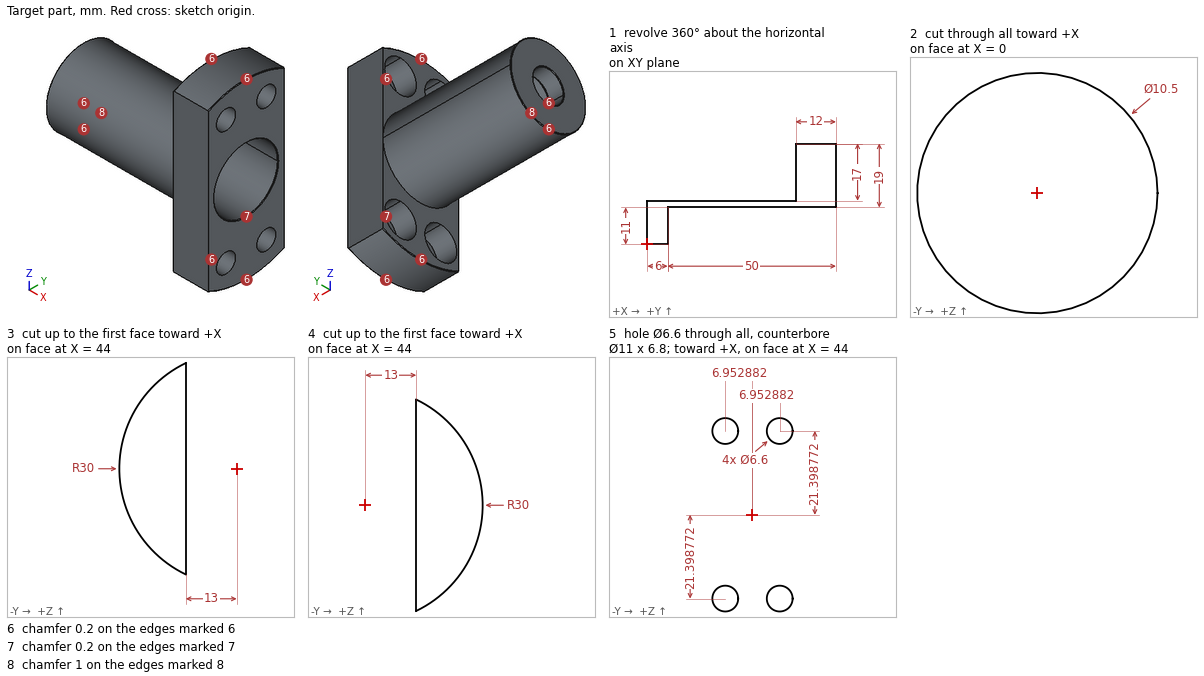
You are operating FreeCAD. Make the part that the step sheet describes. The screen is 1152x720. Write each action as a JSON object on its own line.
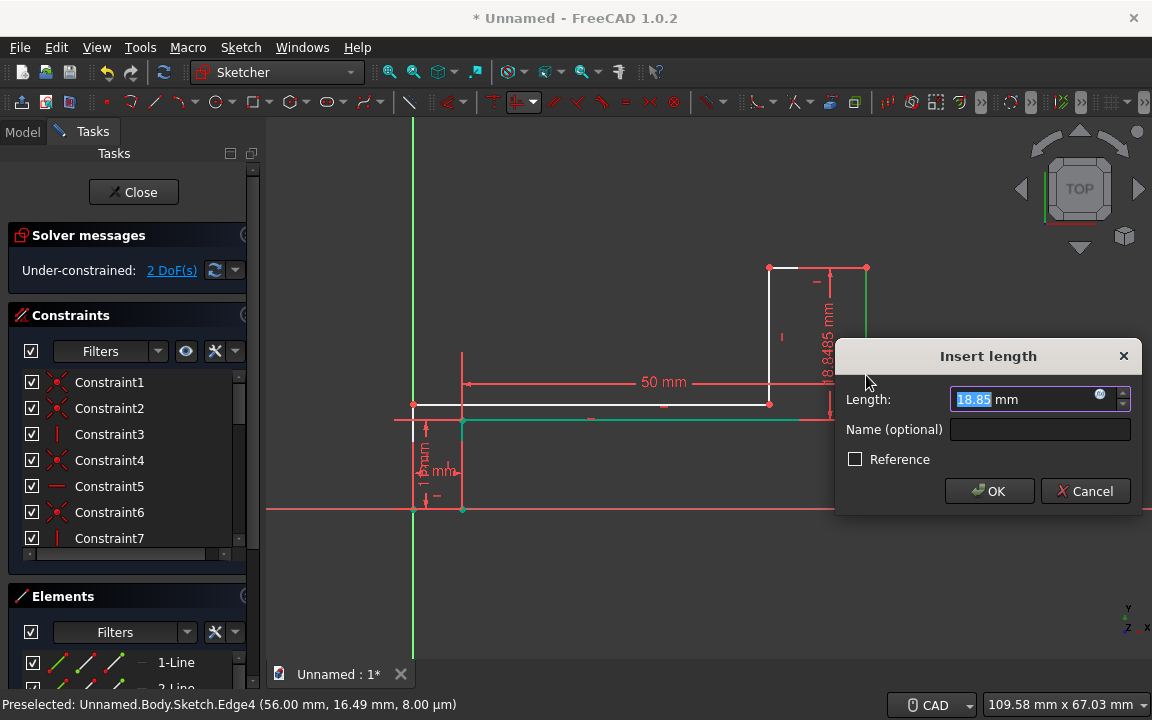
{"action": "type", "text": "19"}
{"action": "key", "text": "Return"}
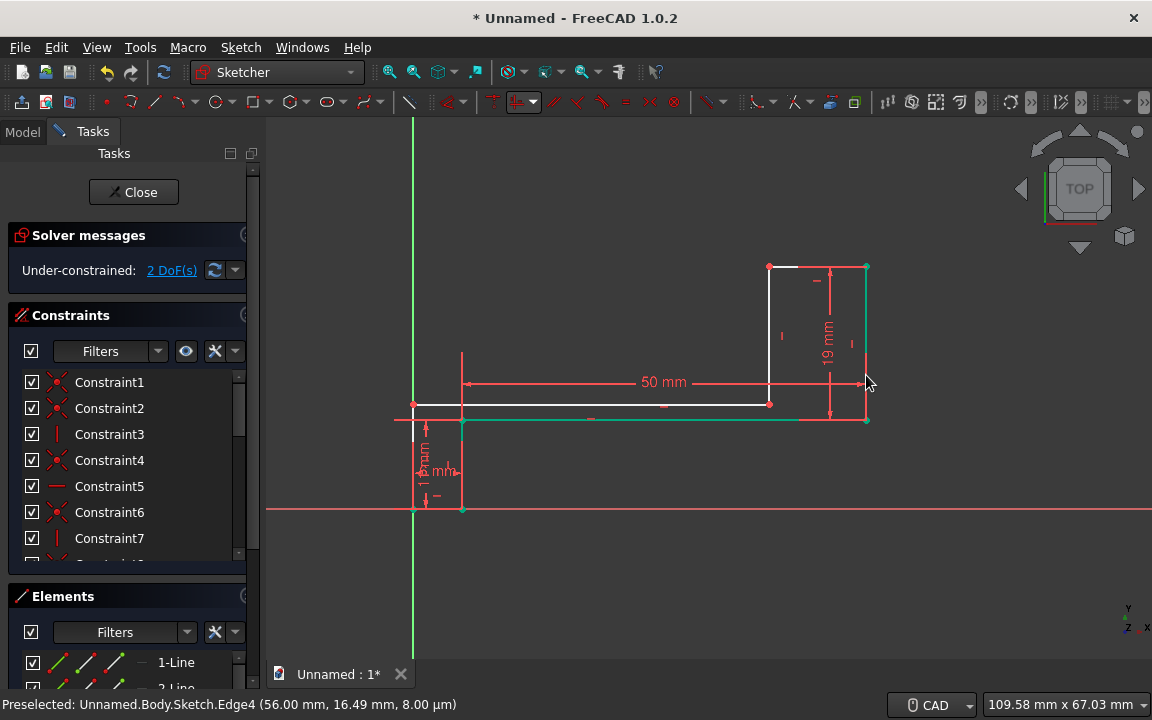
{"action": "left_click", "coordinate": [837, 267]}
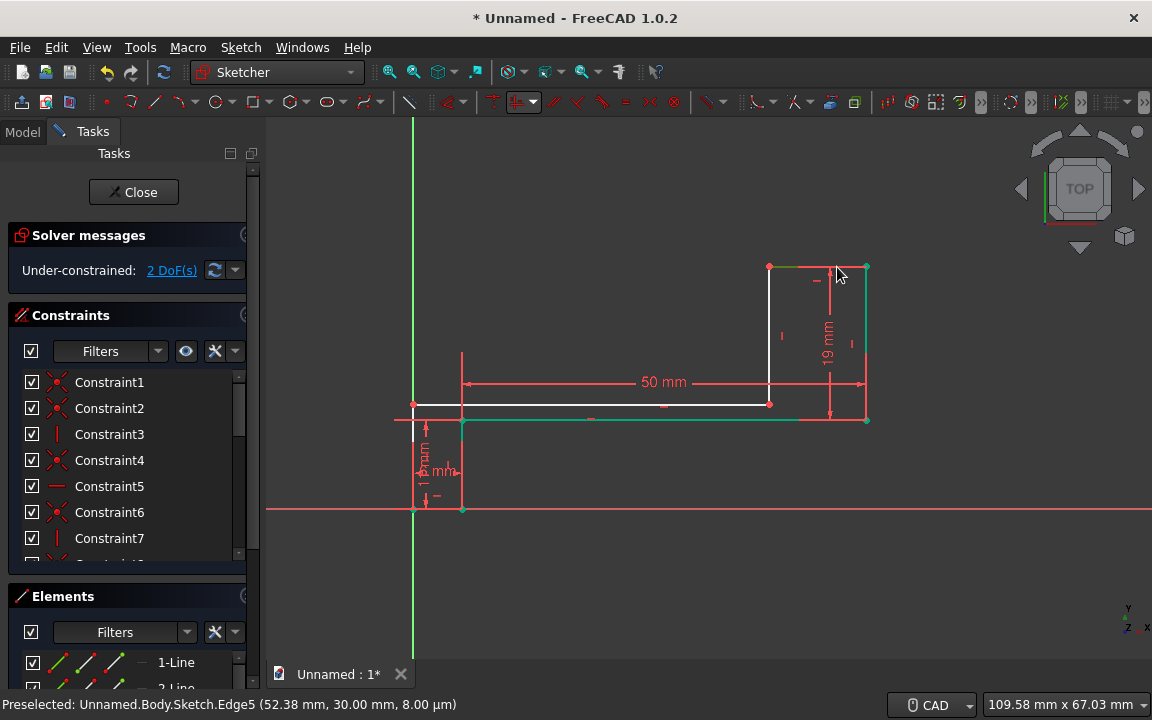
{"action": "key", "text": "l"}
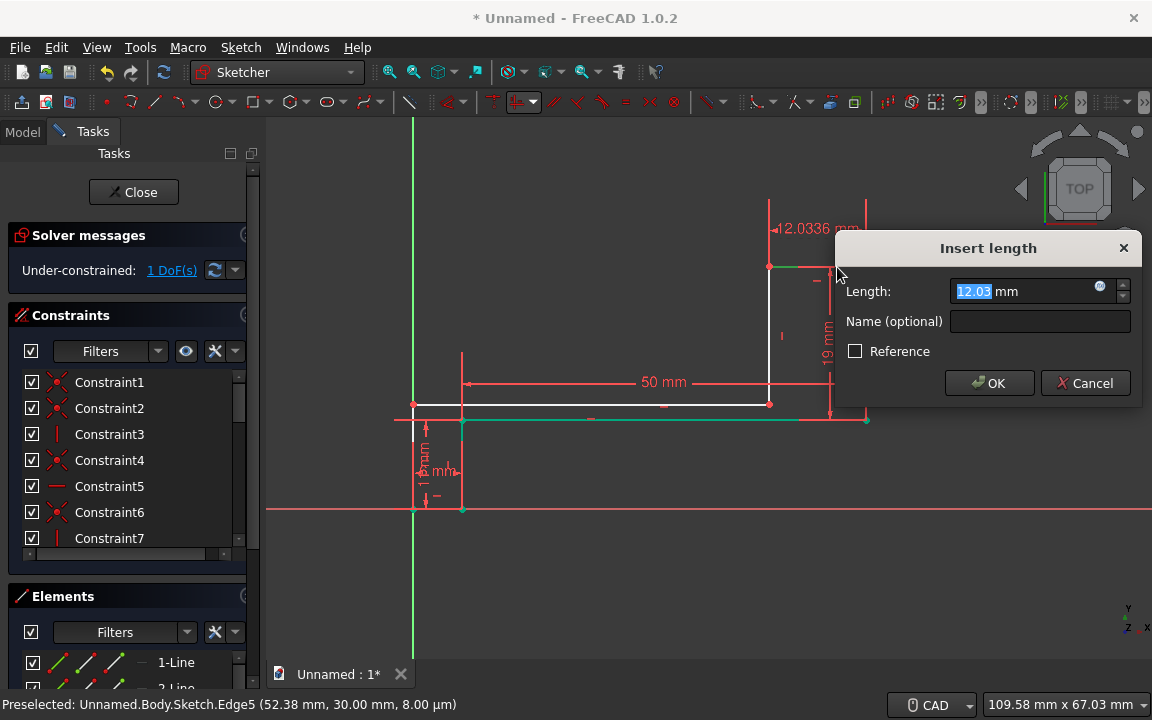
{"action": "type", "text": "12"}
{"action": "key", "text": "Return"}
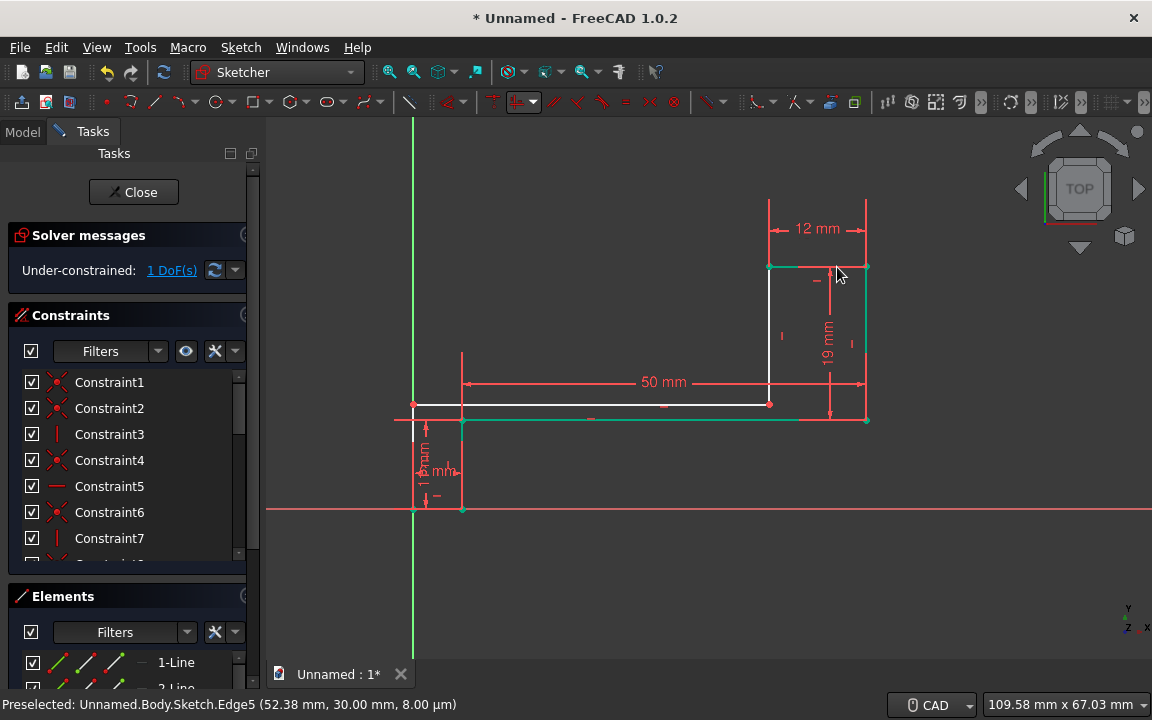
{"action": "left_click", "coordinate": [769, 308]}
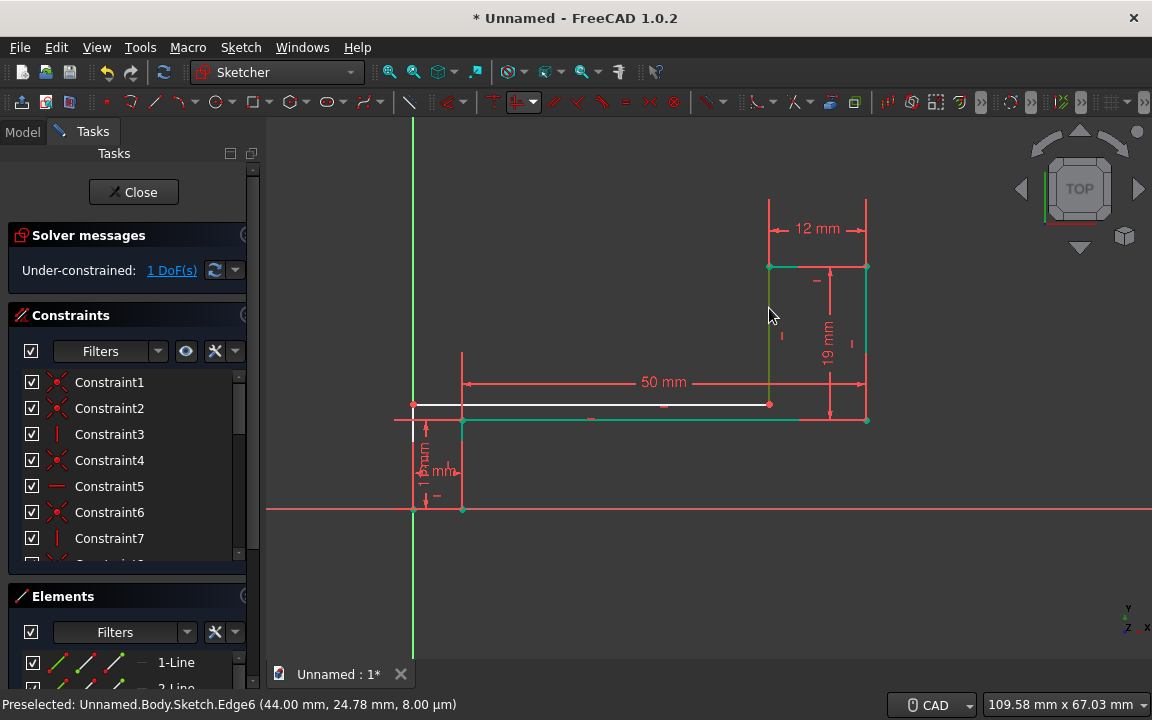
{"action": "key", "text": "i"}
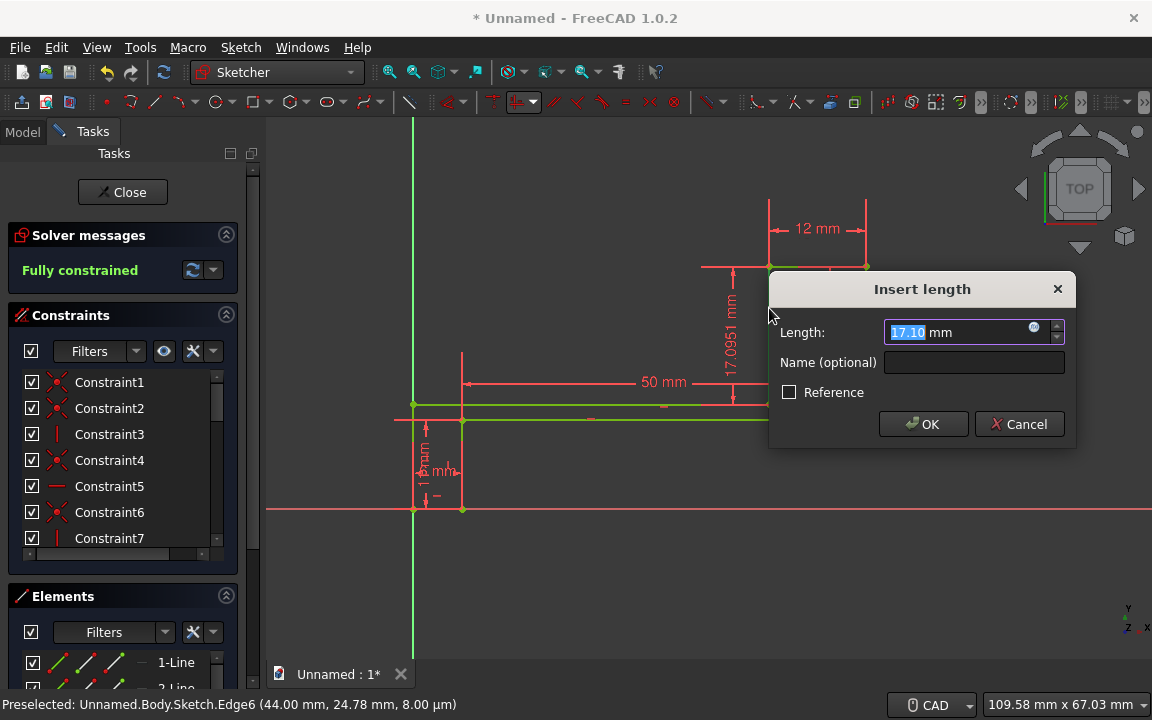
{"action": "type", "text": "17"}
{"action": "key", "text": "Return"}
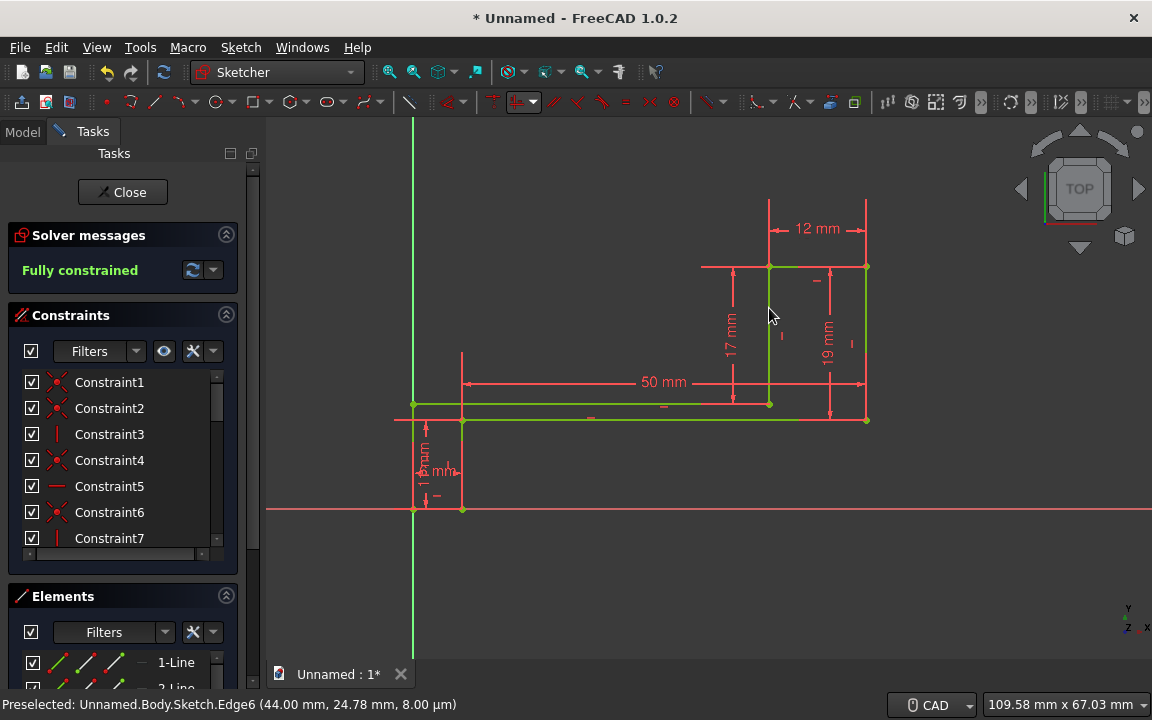
{"action": "left_click", "coordinate": [123, 192]}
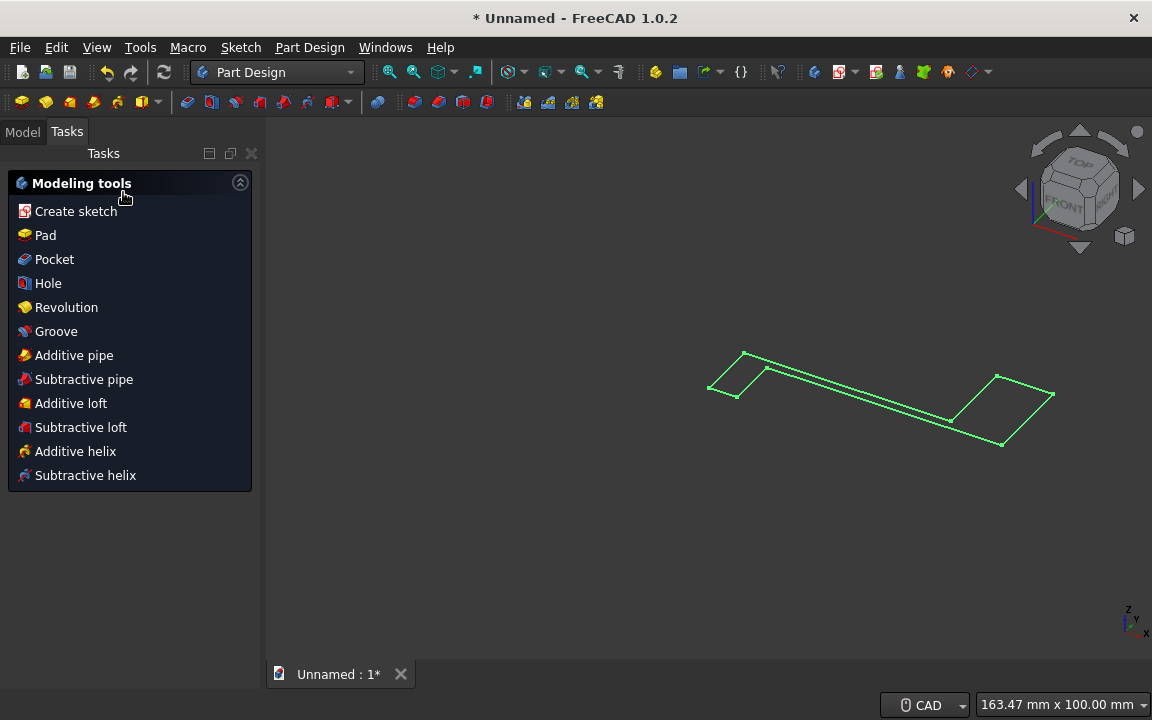
{"action": "left_click", "coordinate": [46, 102]}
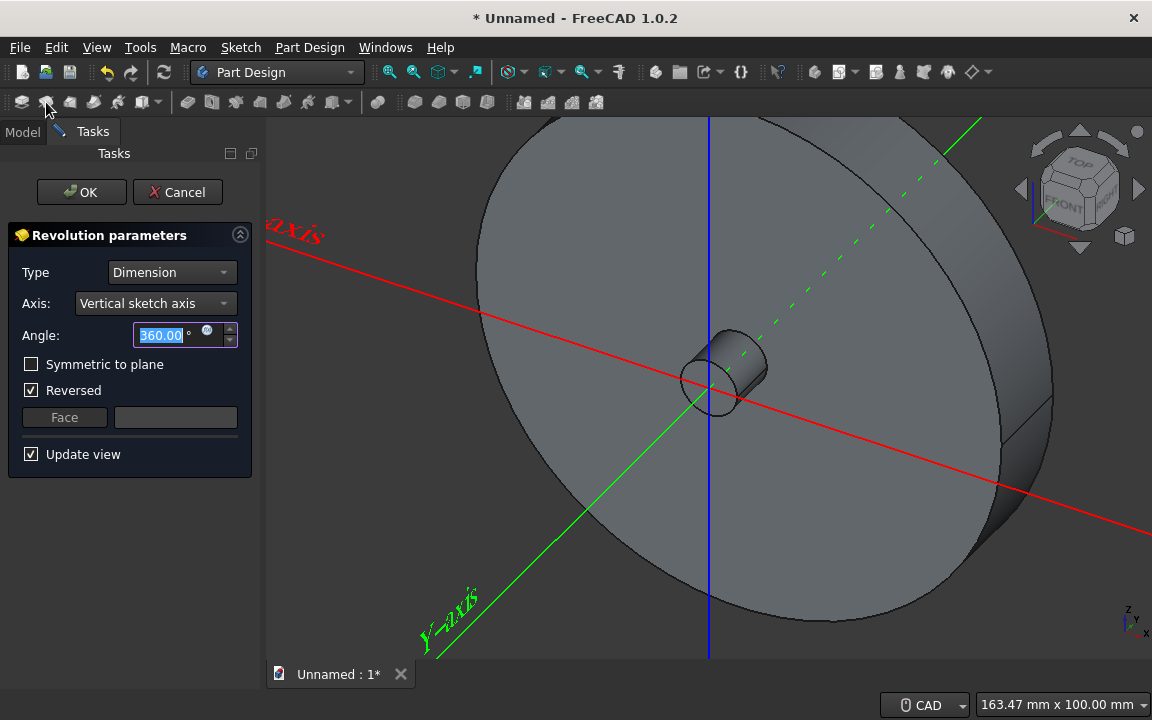
{"action": "left_click", "coordinate": [156, 304]}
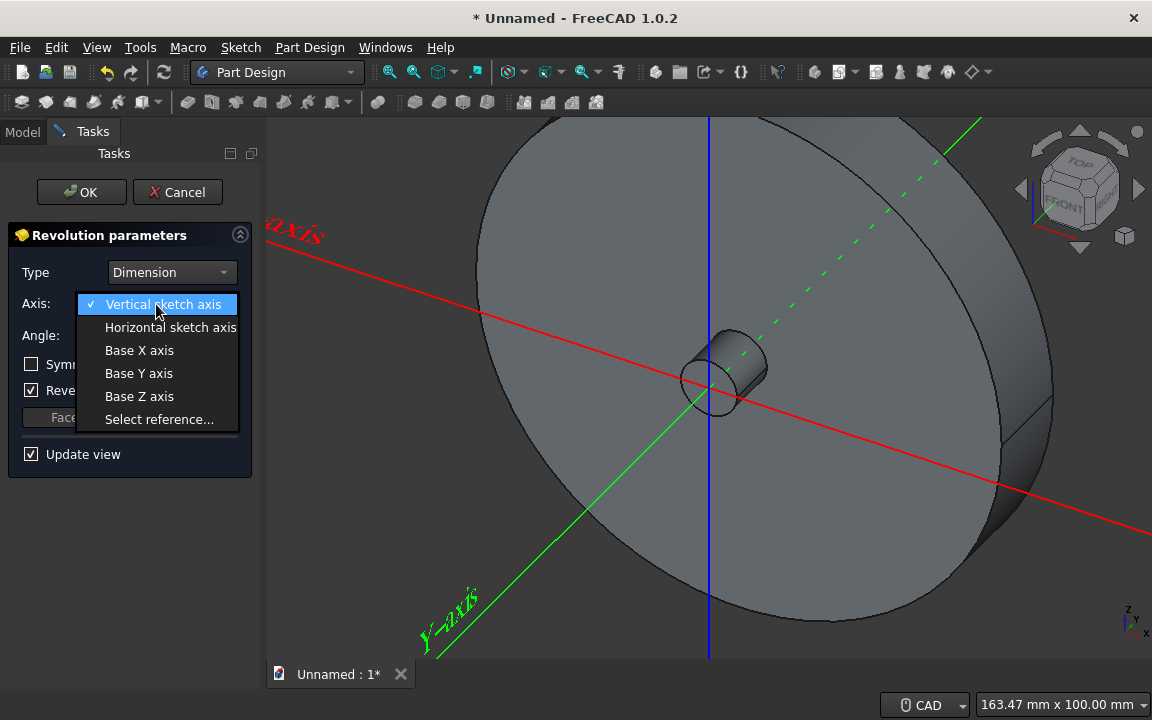
{"action": "left_click", "coordinate": [156, 328]}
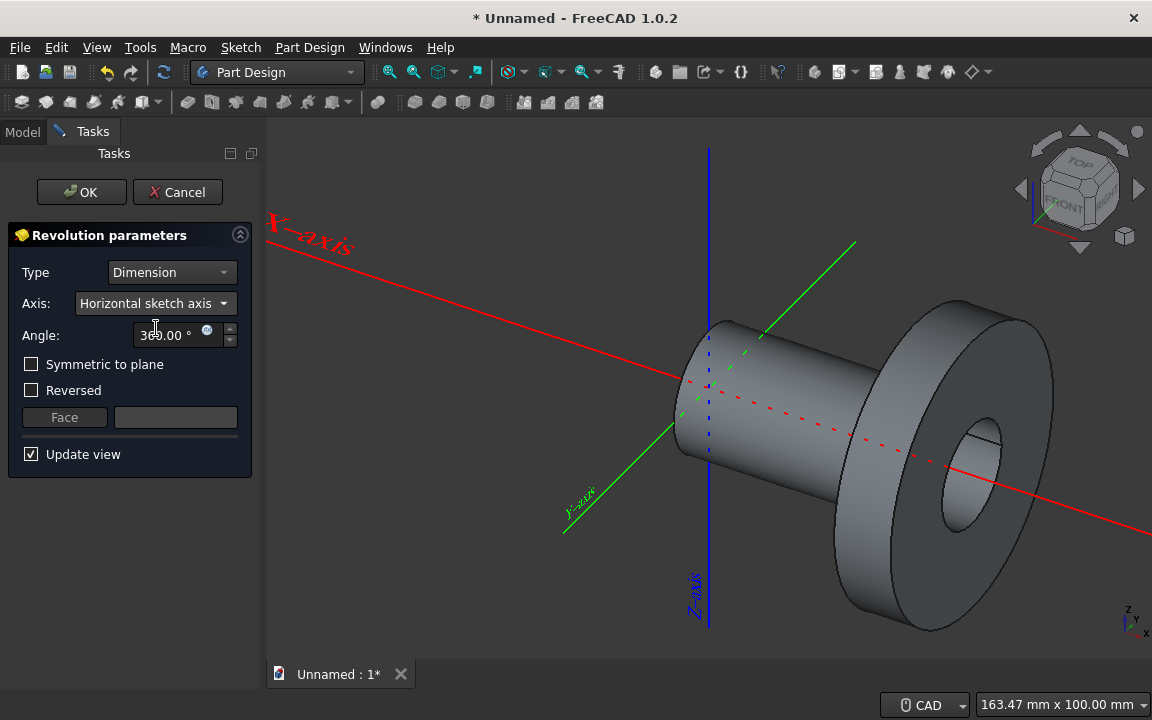
{"action": "left_click", "coordinate": [82, 192]}